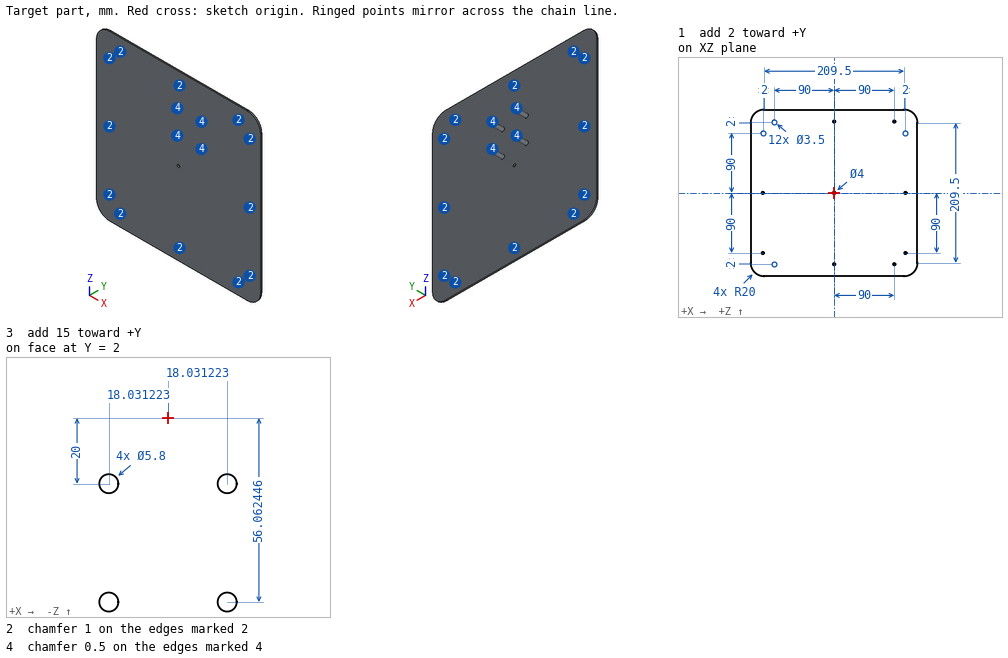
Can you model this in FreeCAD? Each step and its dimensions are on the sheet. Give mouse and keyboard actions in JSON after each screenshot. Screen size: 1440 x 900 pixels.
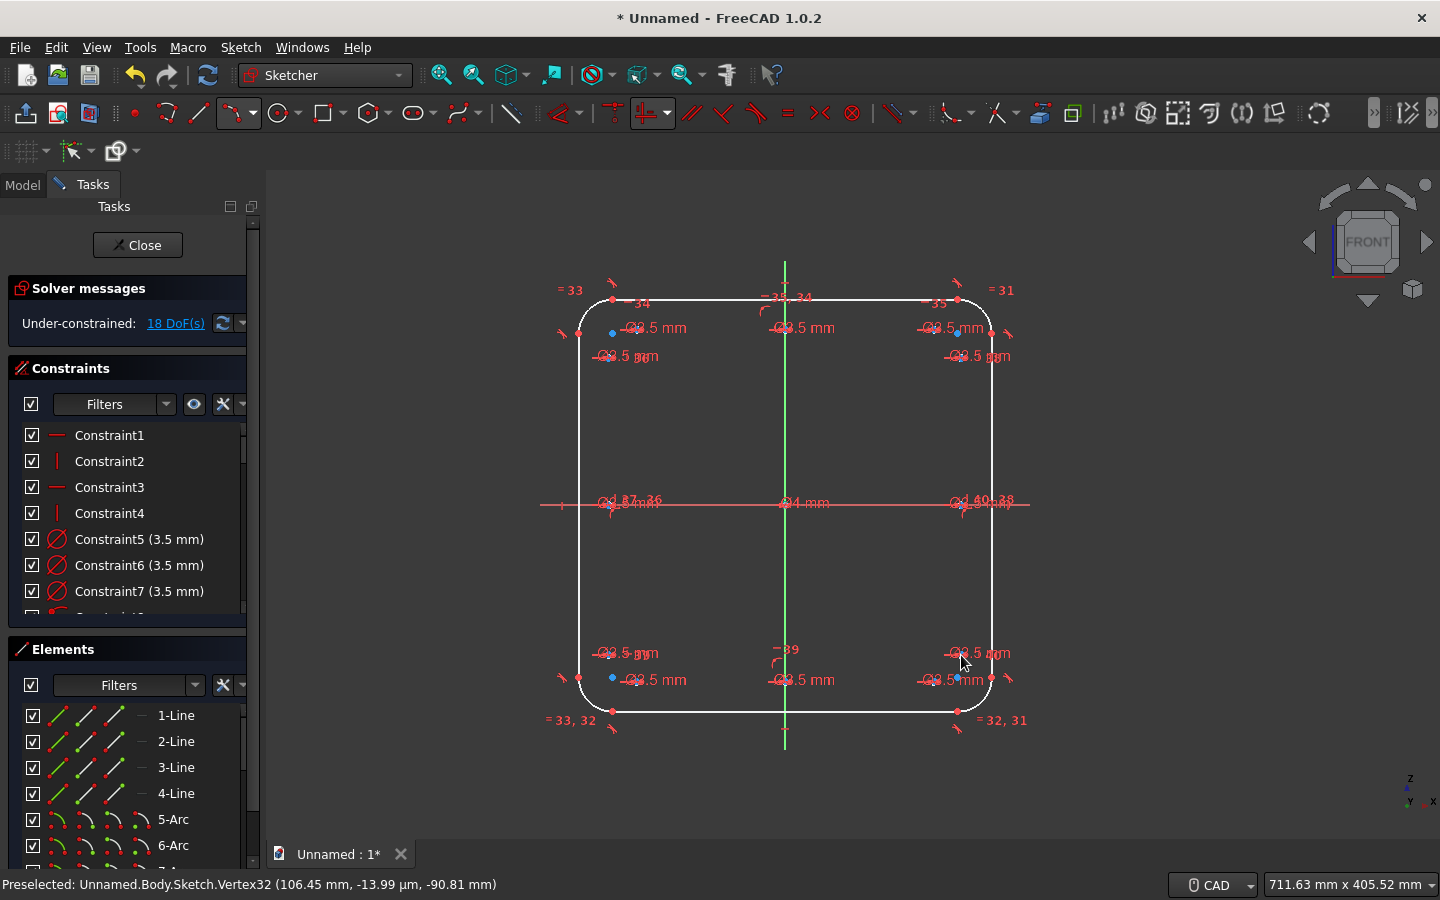
{"action": "left_click", "coordinate": [785, 682]}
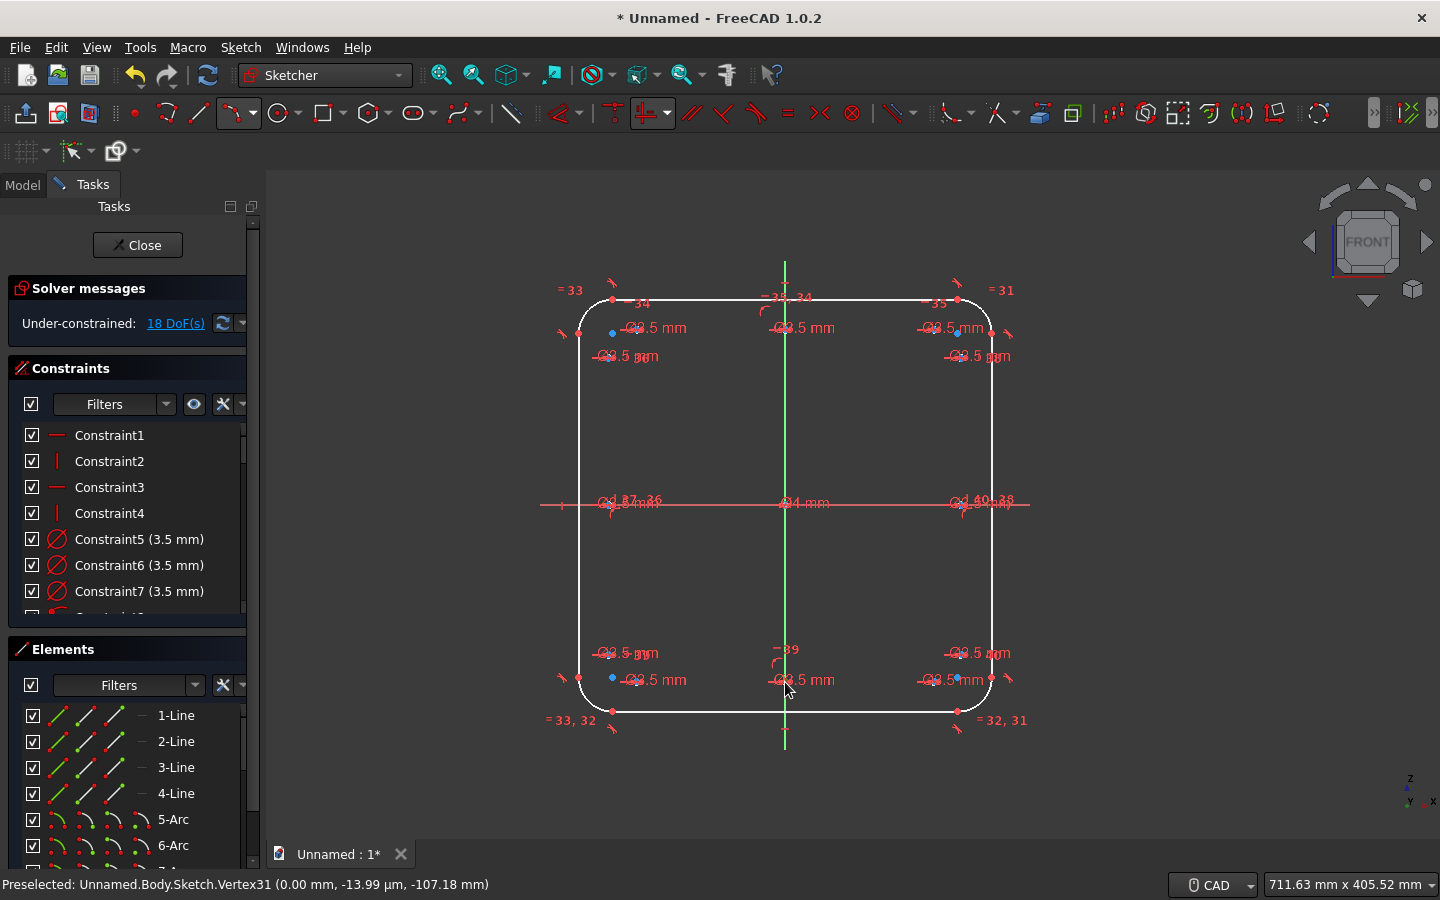
{"action": "left_click", "coordinate": [934, 682]}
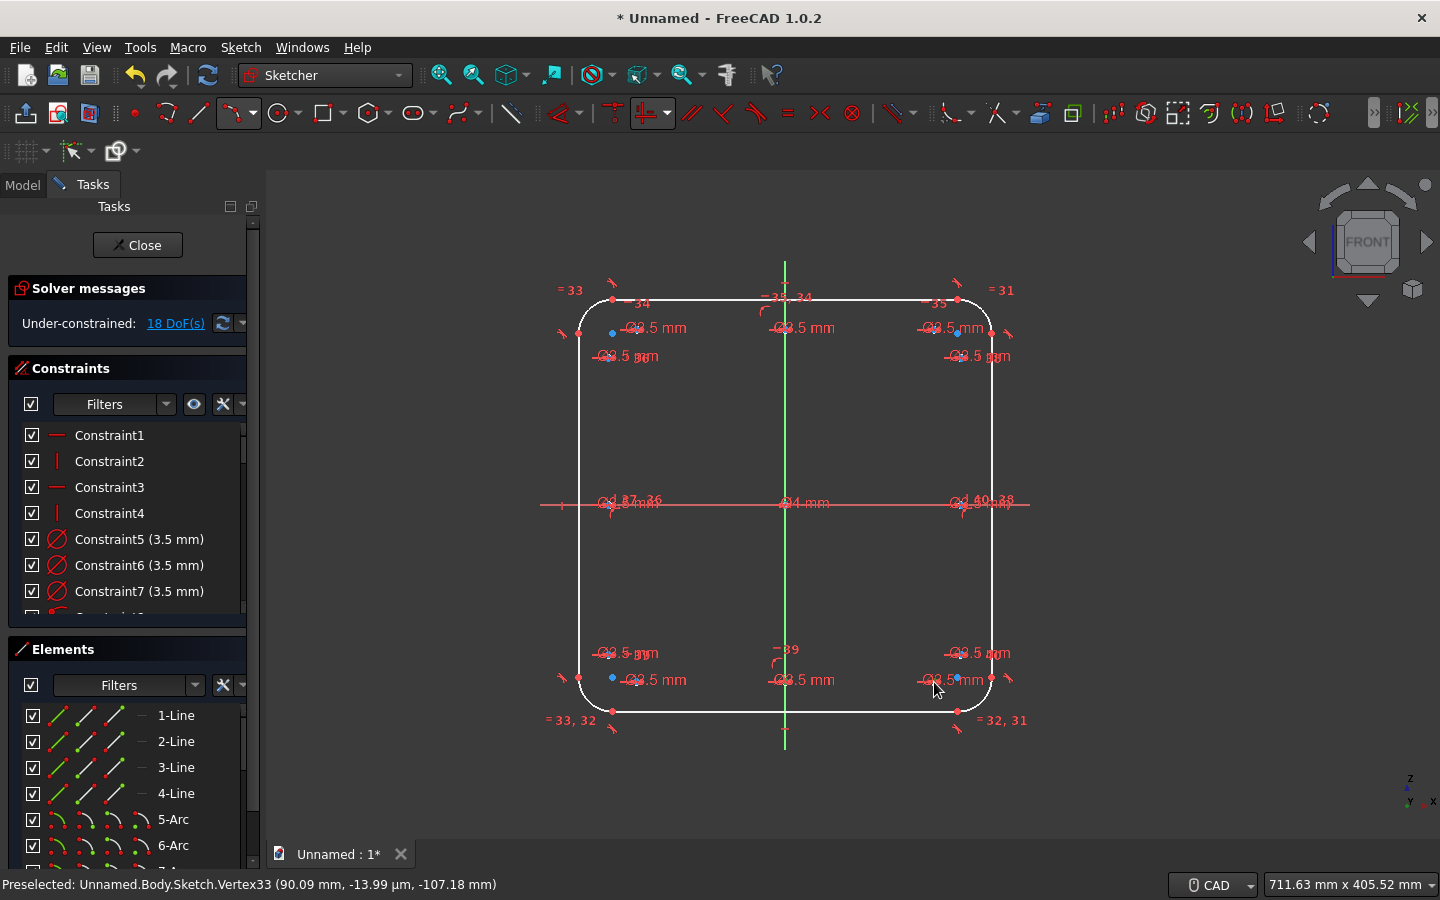
{"action": "key", "text": "h"}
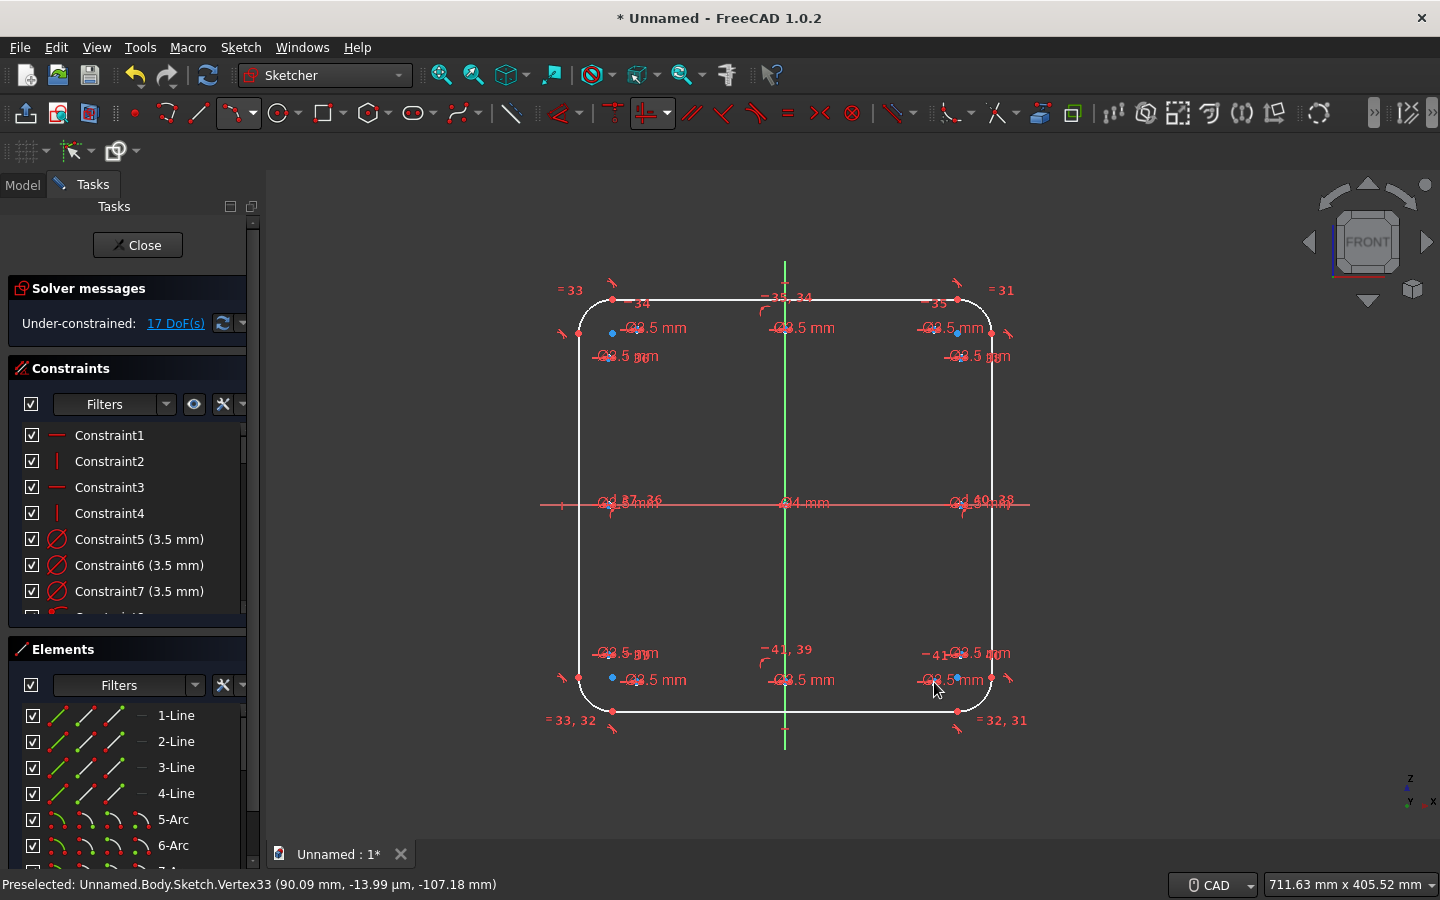
{"action": "left_click", "coordinate": [609, 358]}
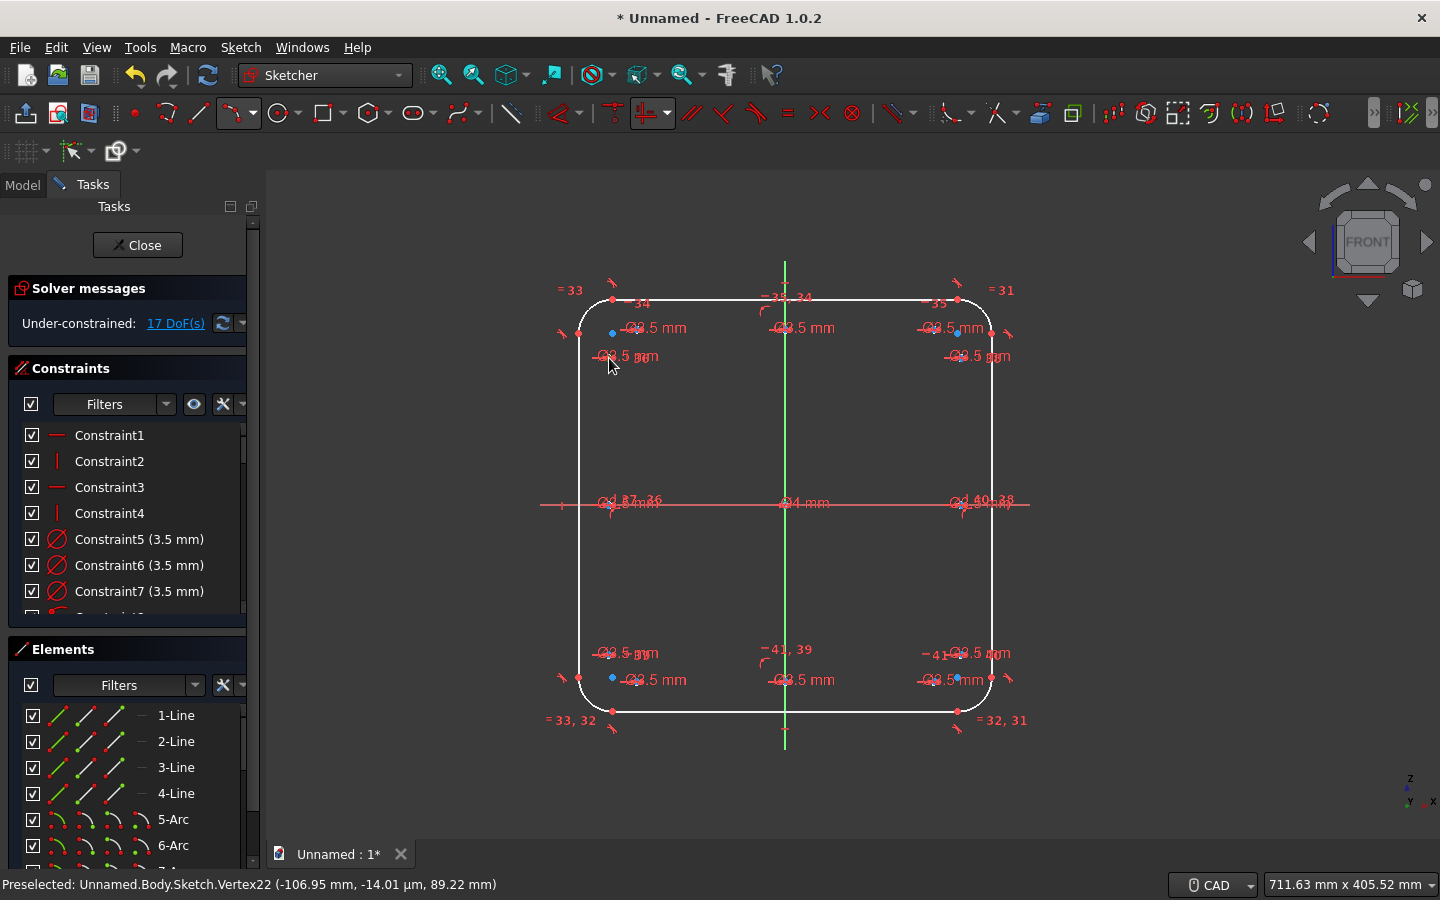
{"action": "left_click", "coordinate": [961, 358]}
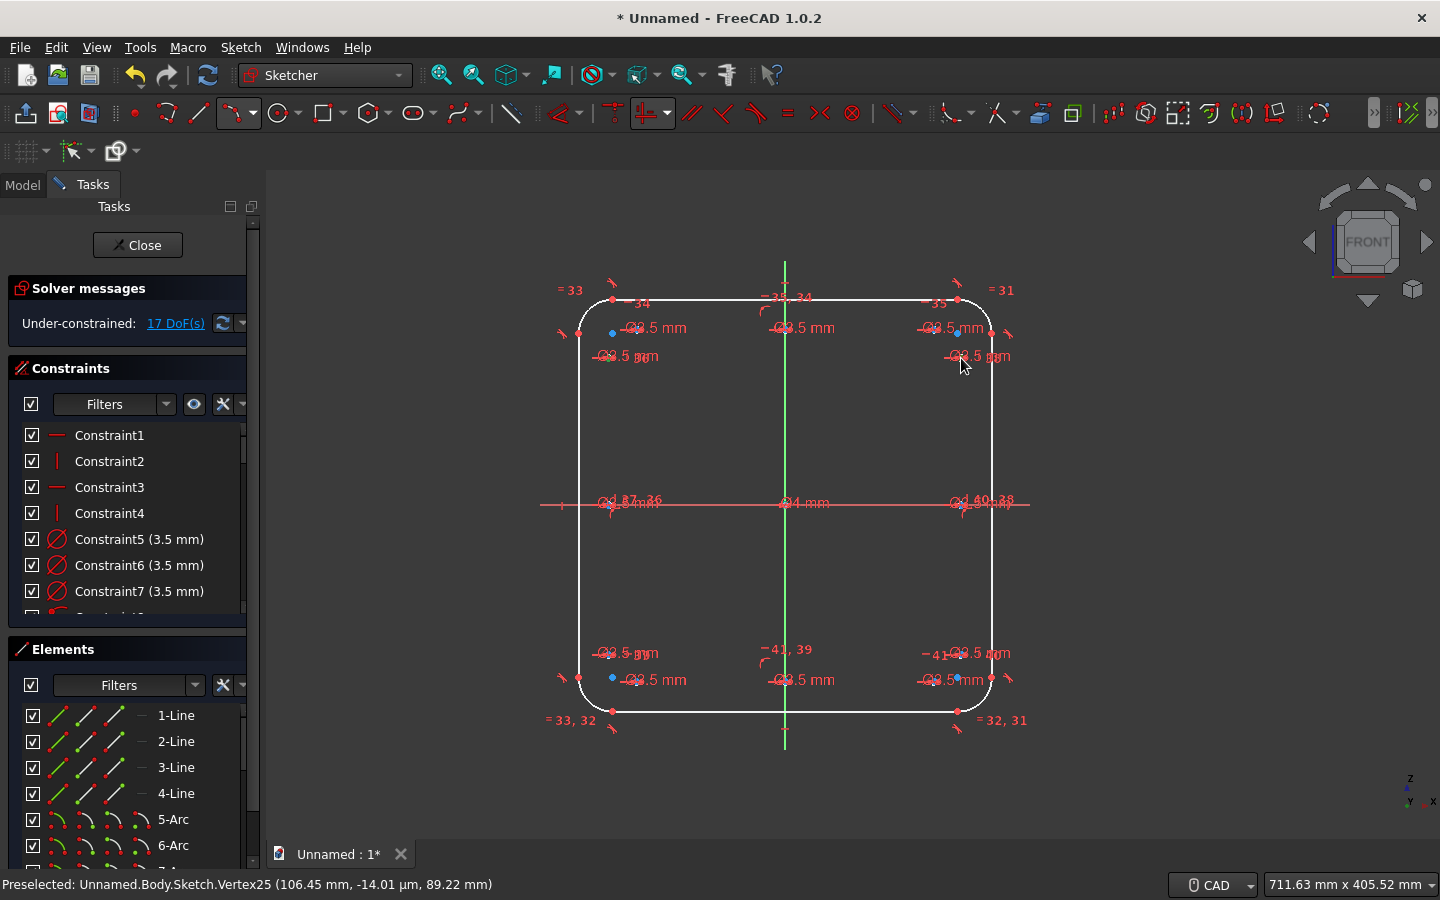
{"action": "left_click", "coordinate": [785, 636]}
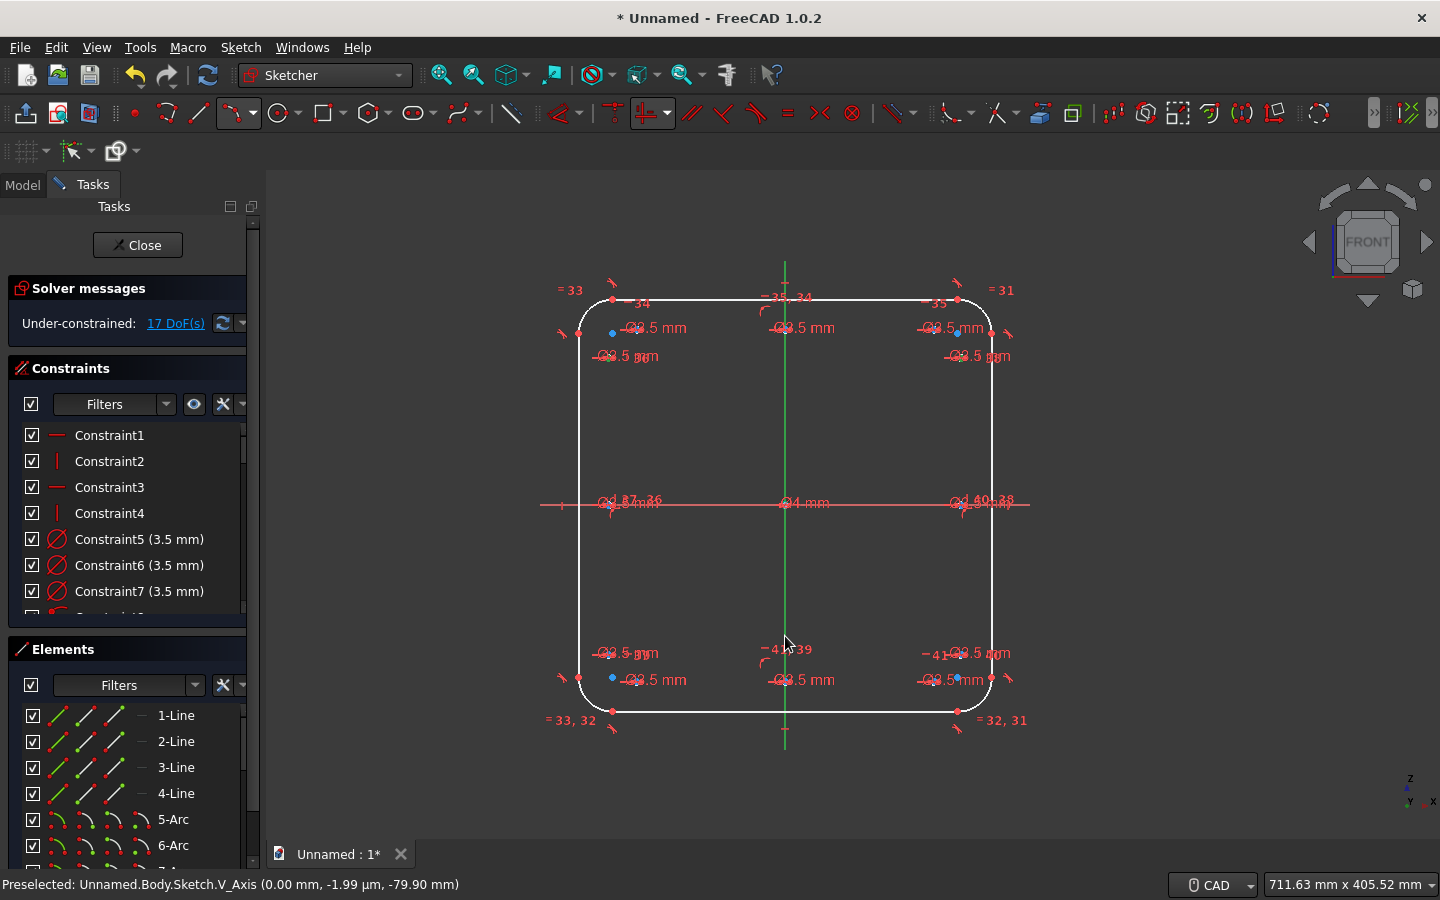
{"action": "key", "text": "s"}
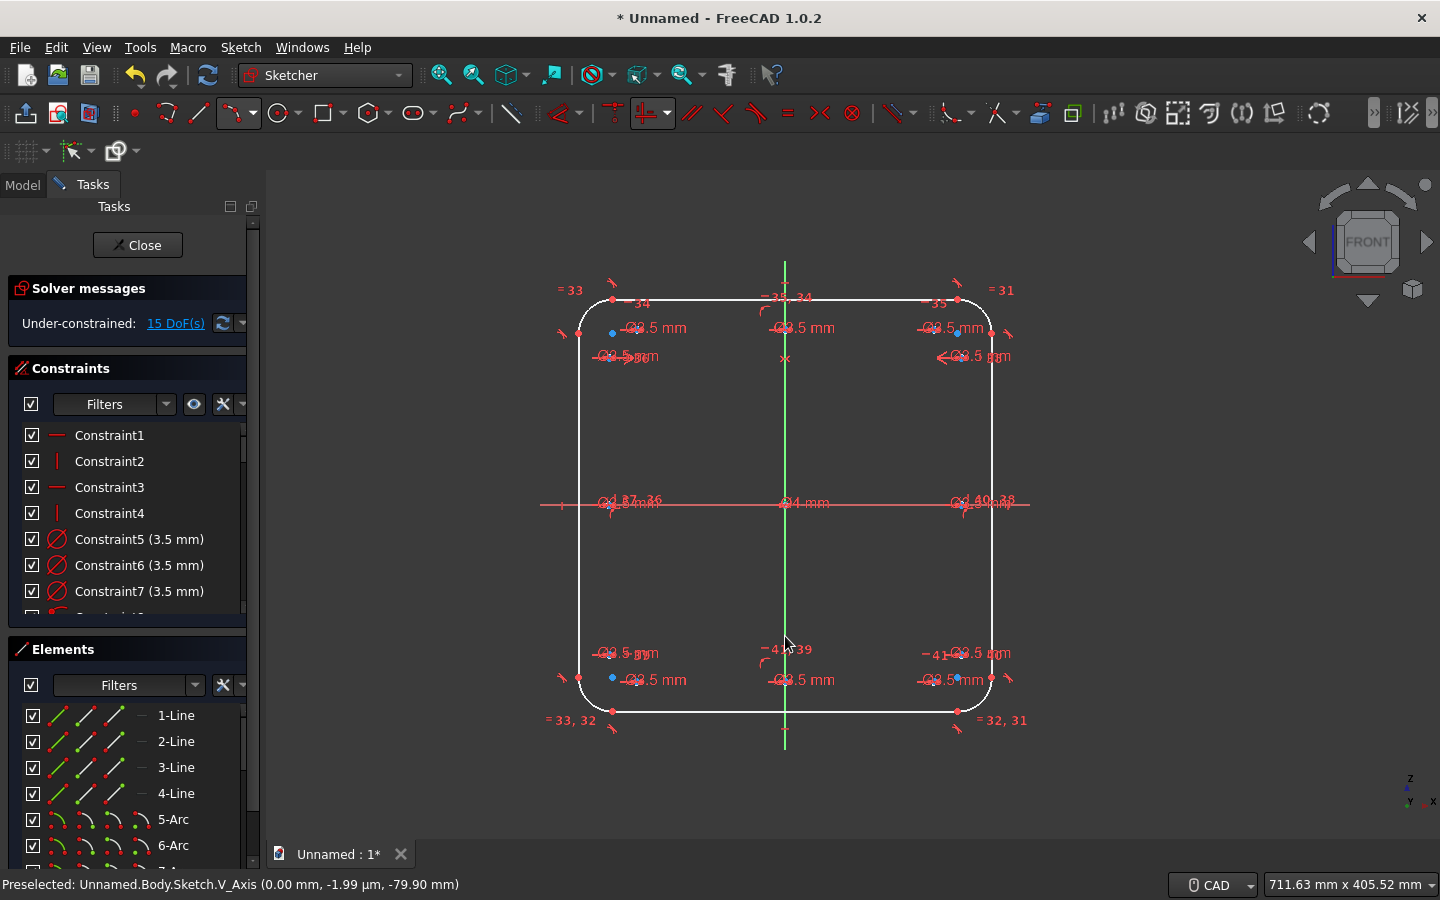
{"action": "left_click", "coordinate": [637, 330]}